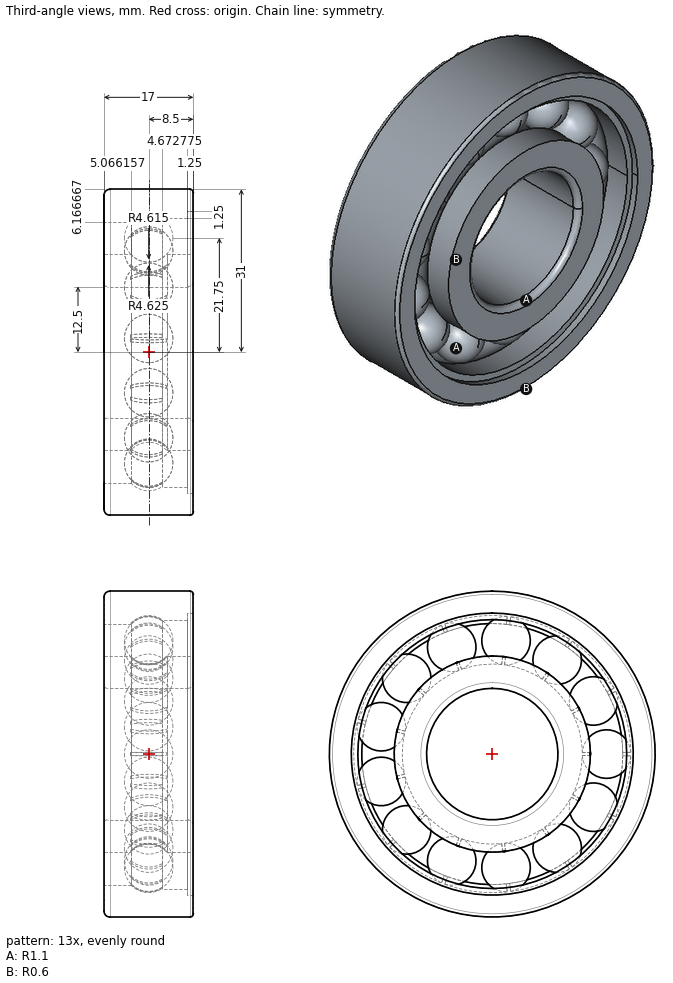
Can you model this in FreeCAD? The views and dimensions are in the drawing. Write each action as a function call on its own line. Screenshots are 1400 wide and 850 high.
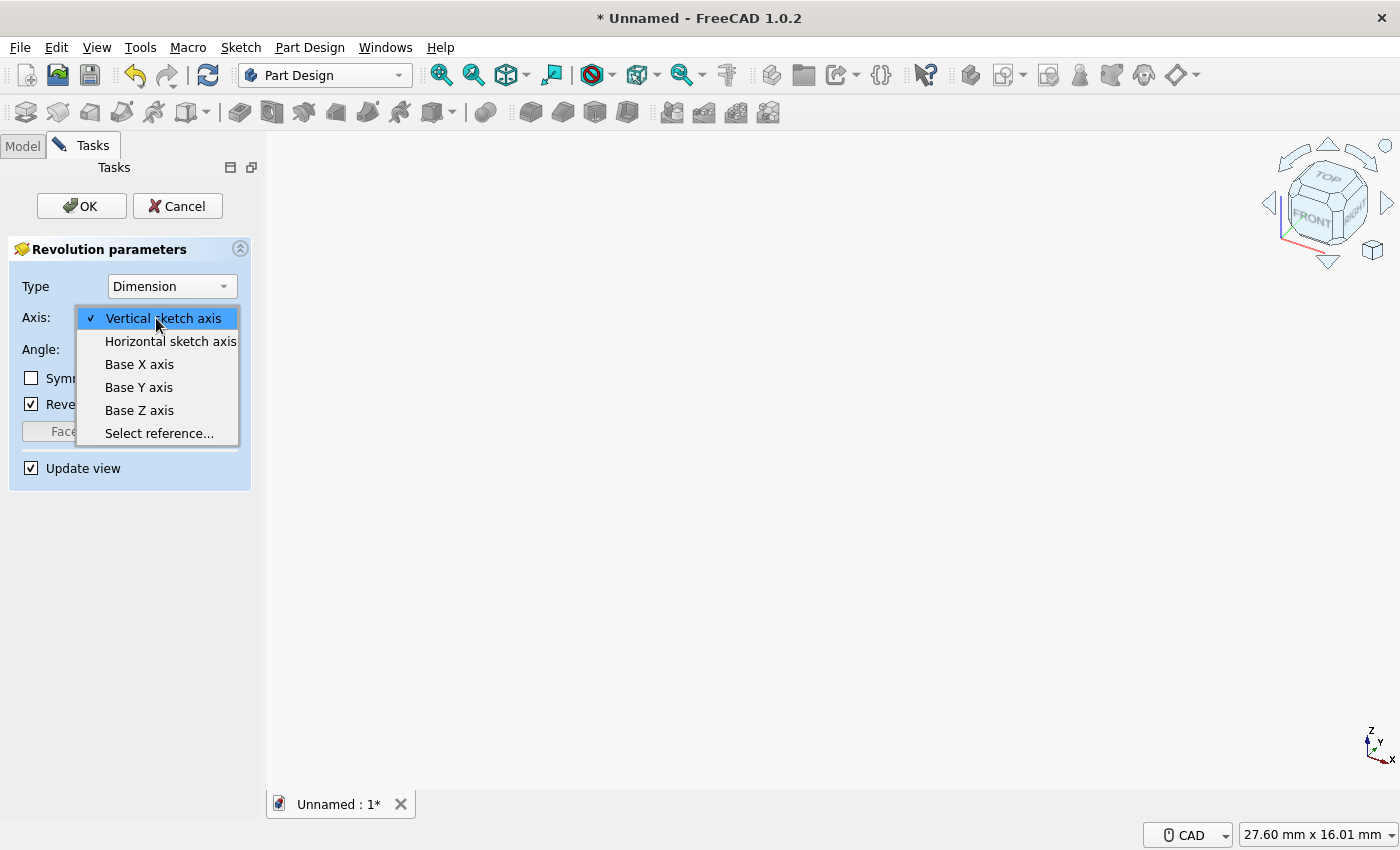
click(156, 342)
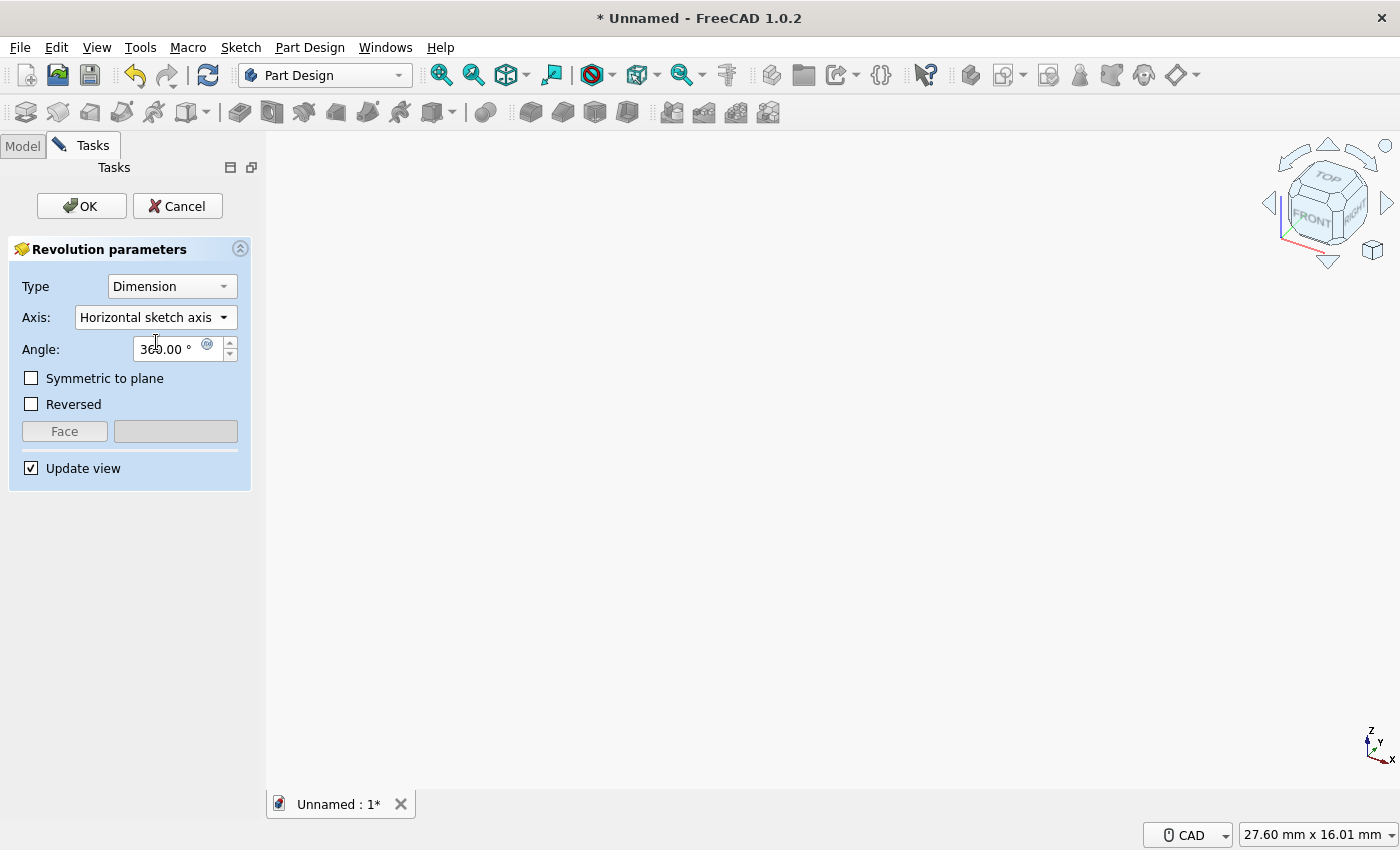
click(82, 206)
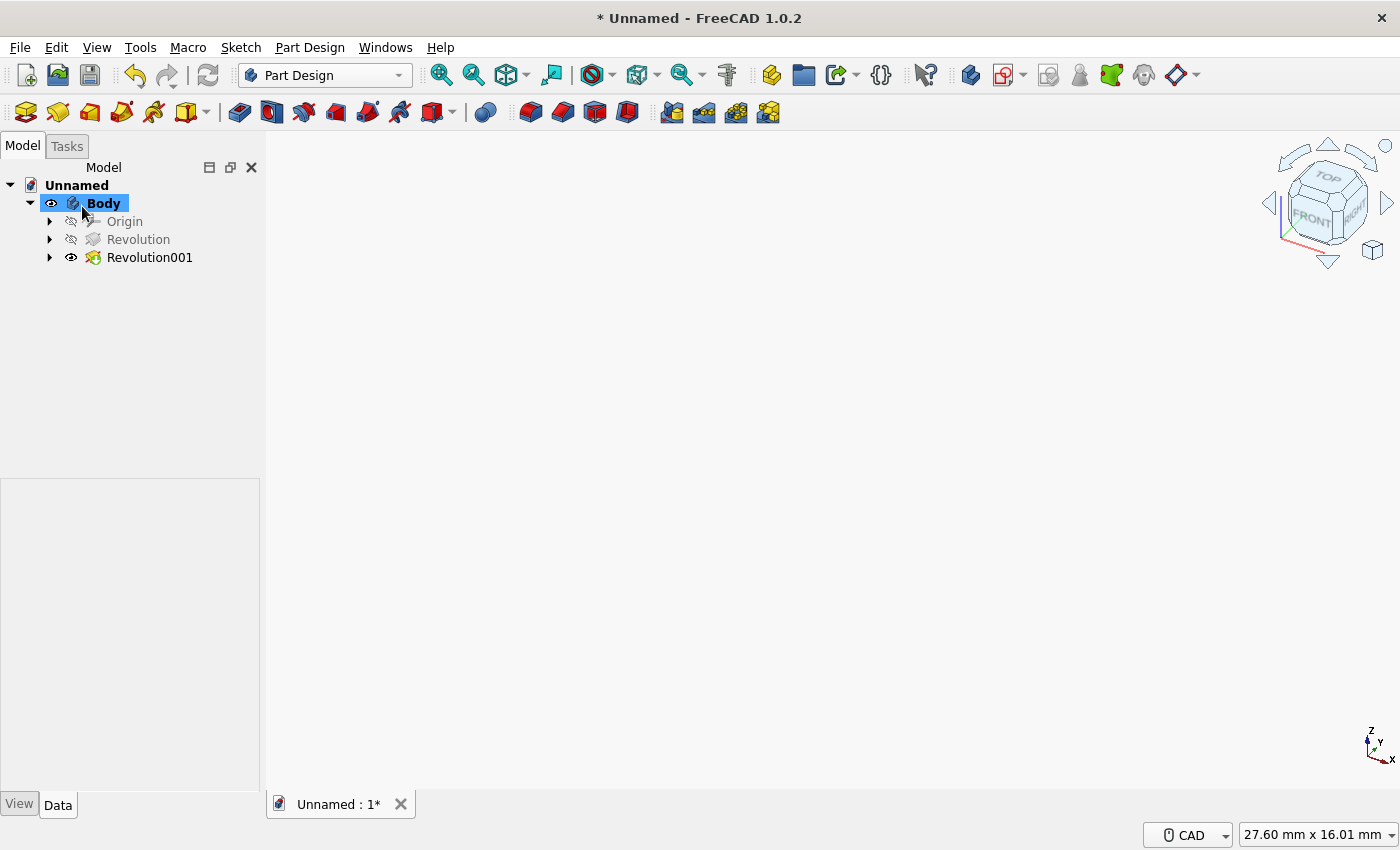
click(442, 76)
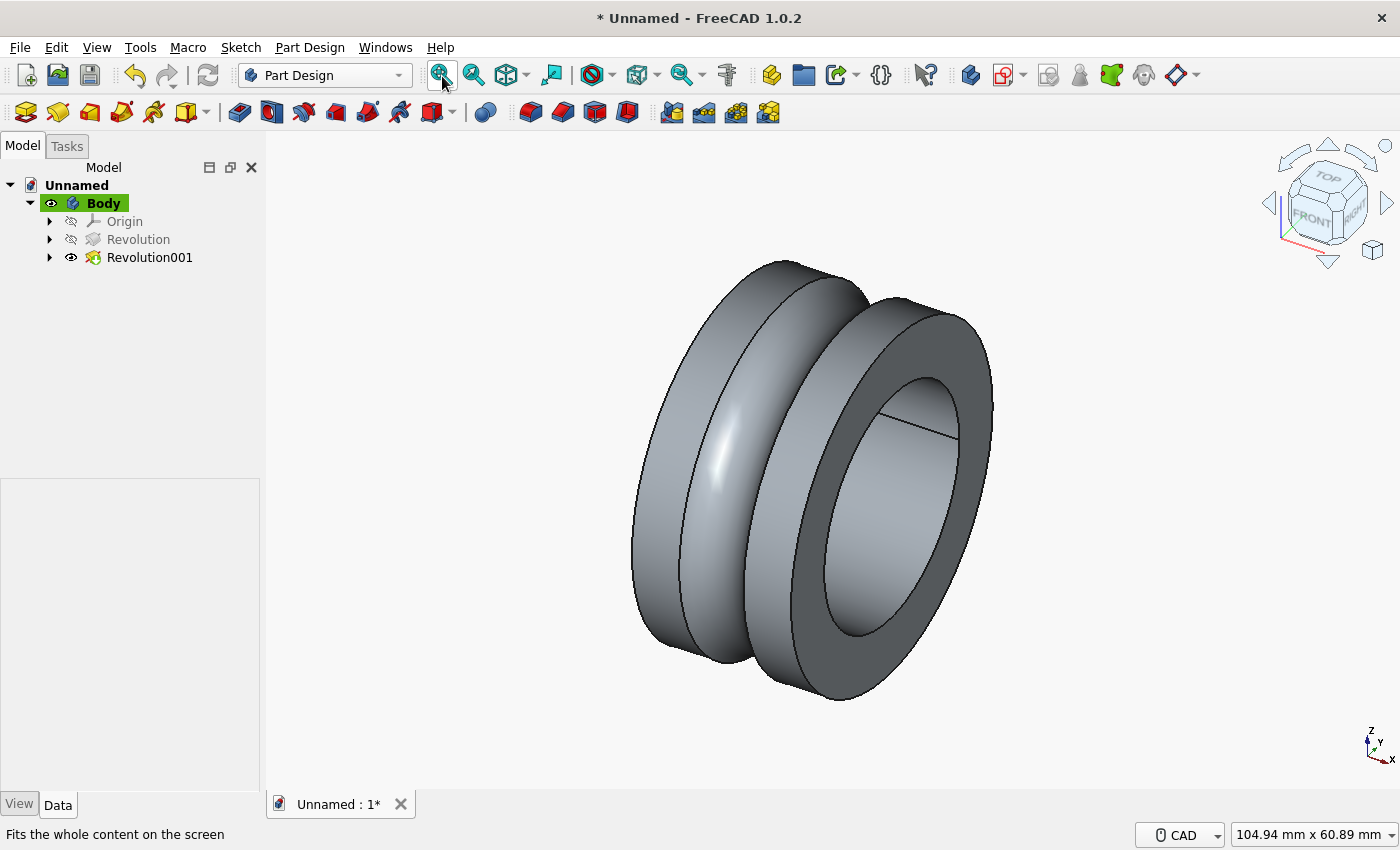
click(1004, 76)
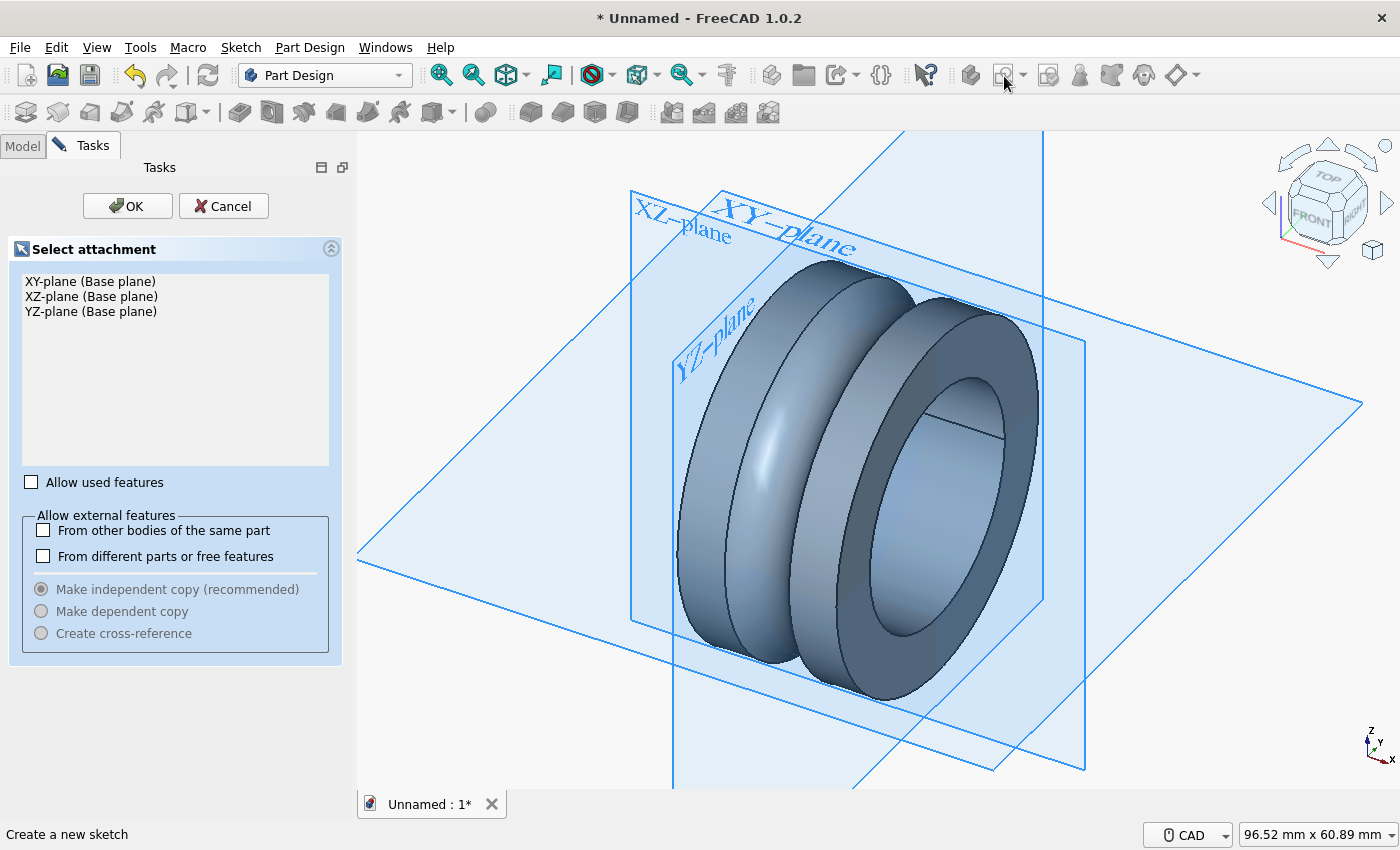
click(82, 282)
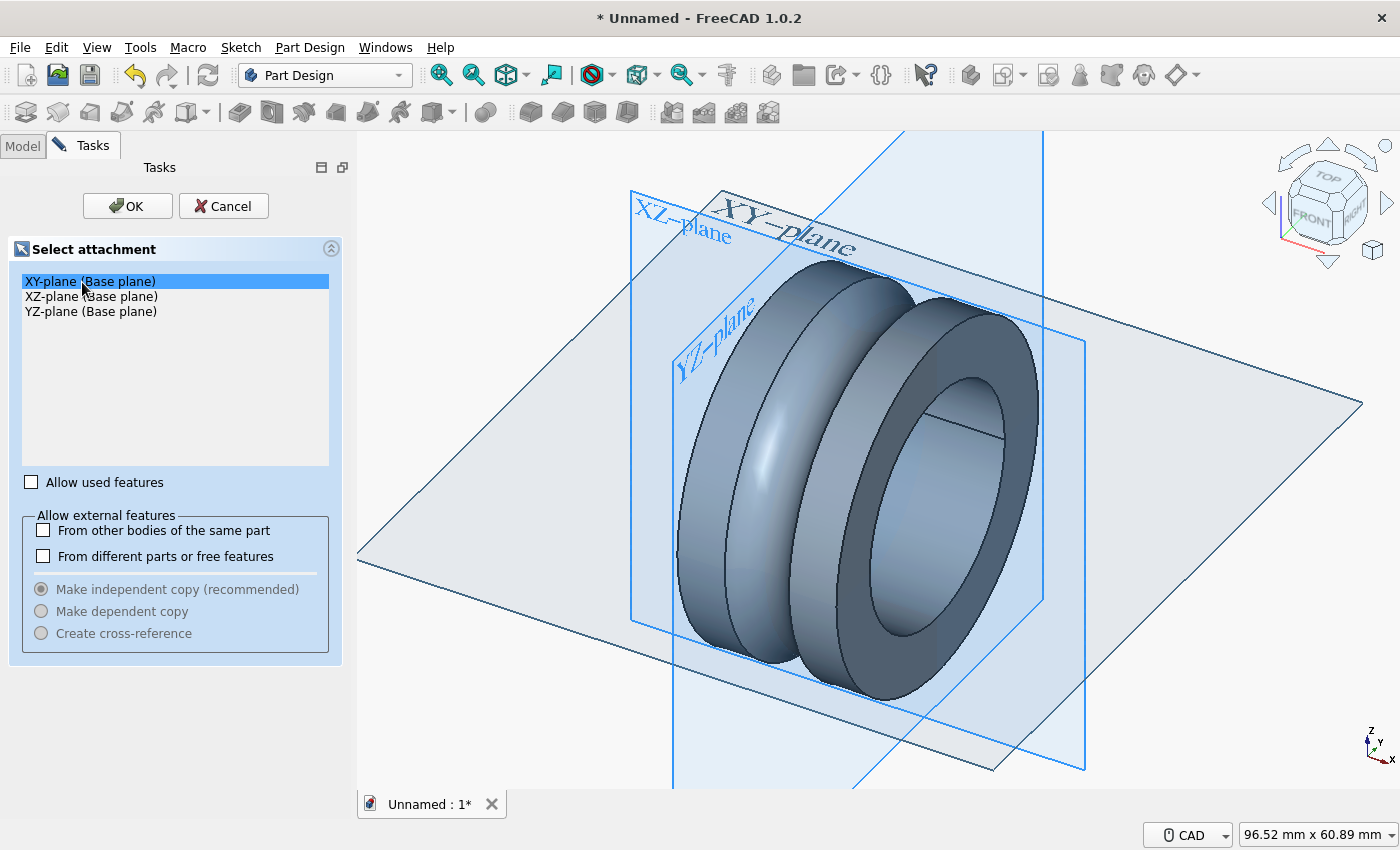
click(128, 206)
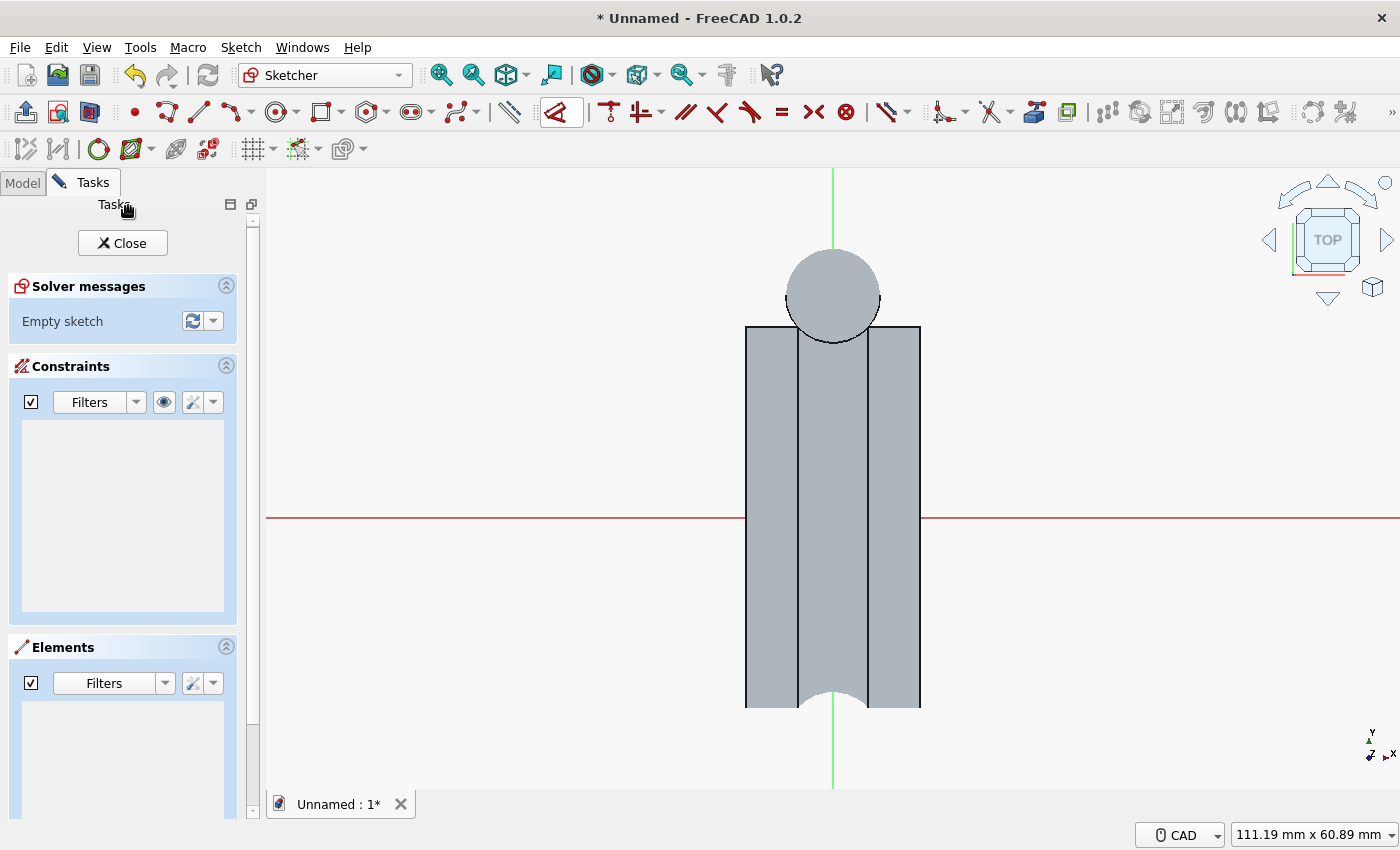
click(90, 112)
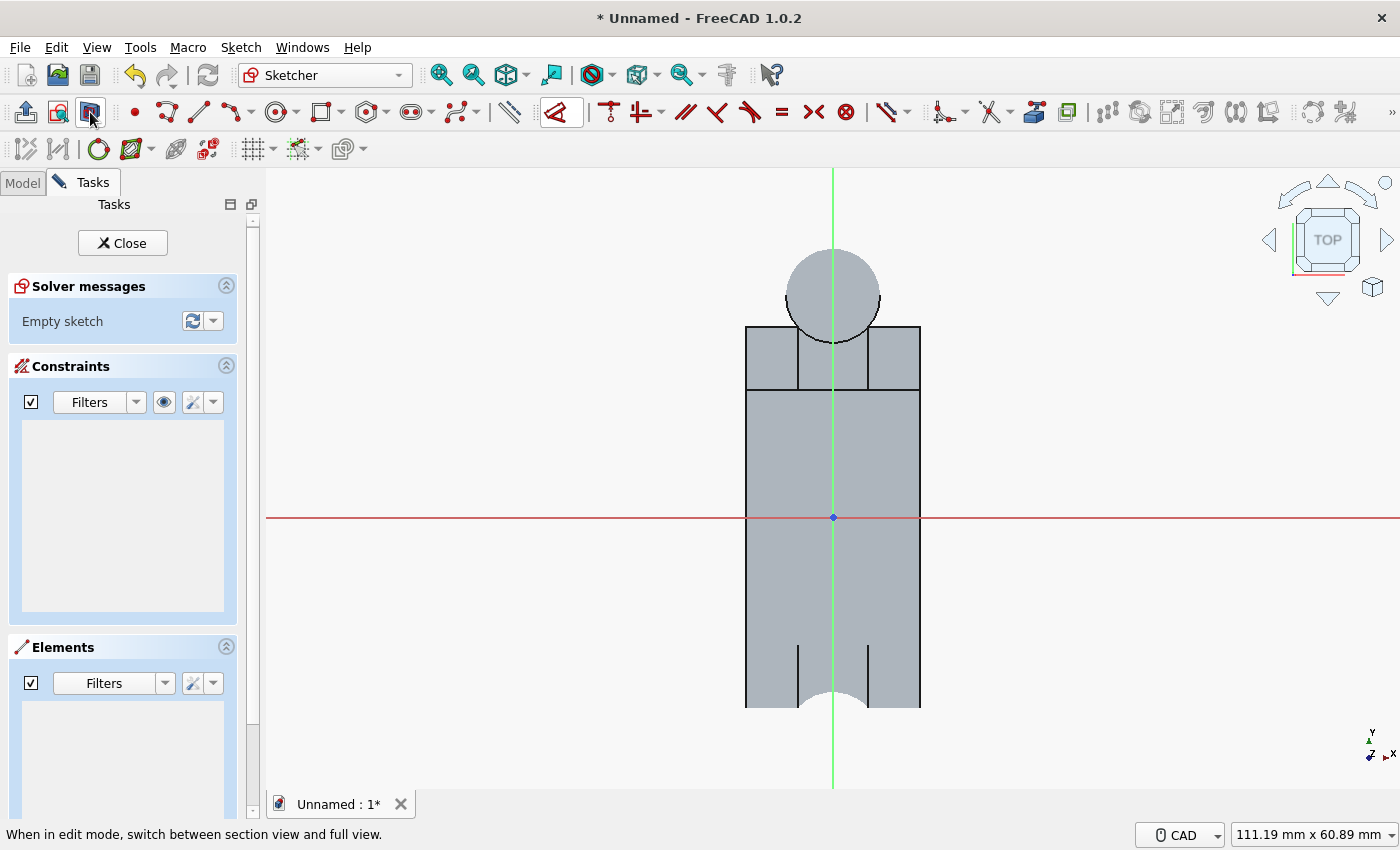
scroll(455, 761, down, 1)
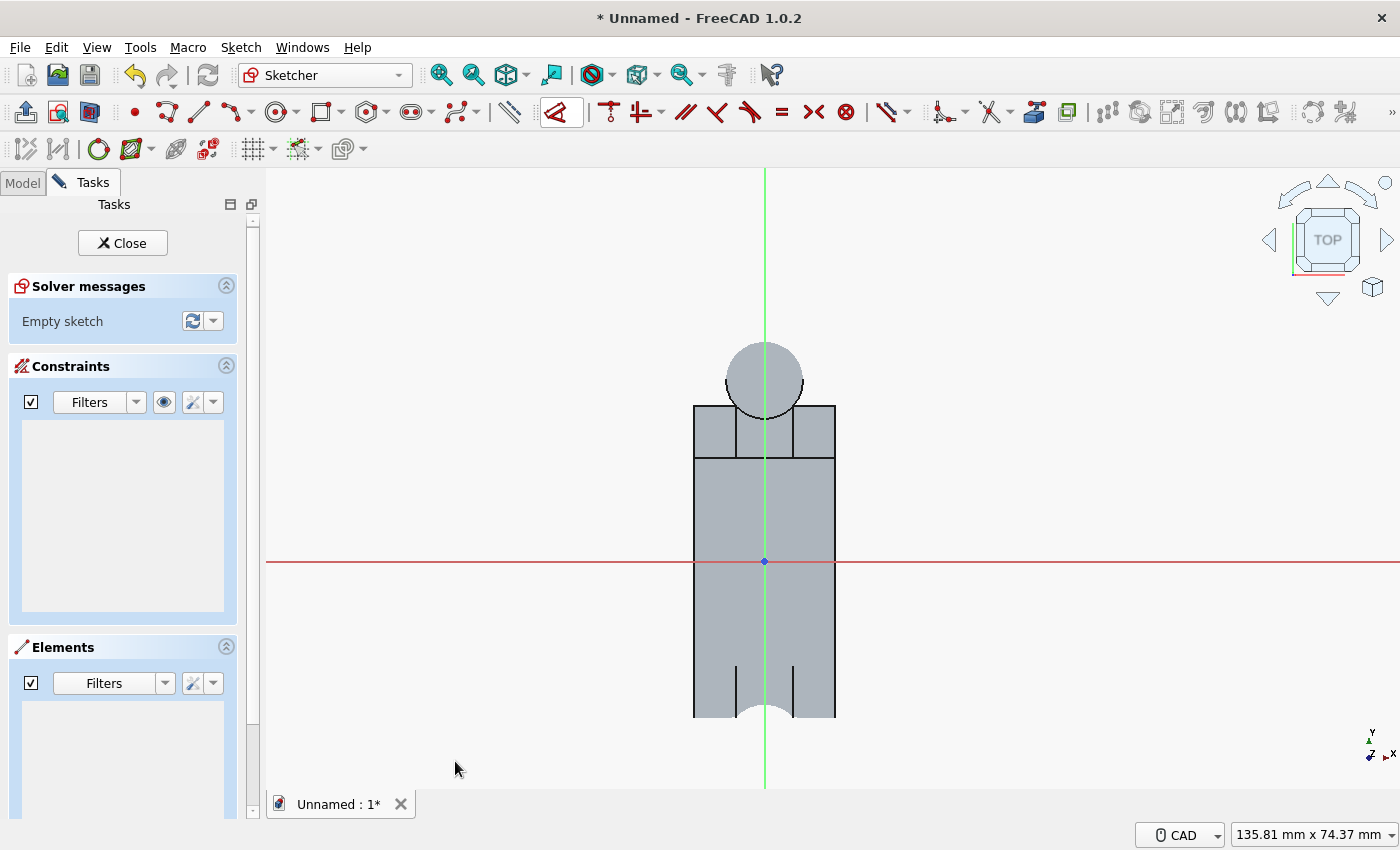
scroll(765, 339, up, 2)